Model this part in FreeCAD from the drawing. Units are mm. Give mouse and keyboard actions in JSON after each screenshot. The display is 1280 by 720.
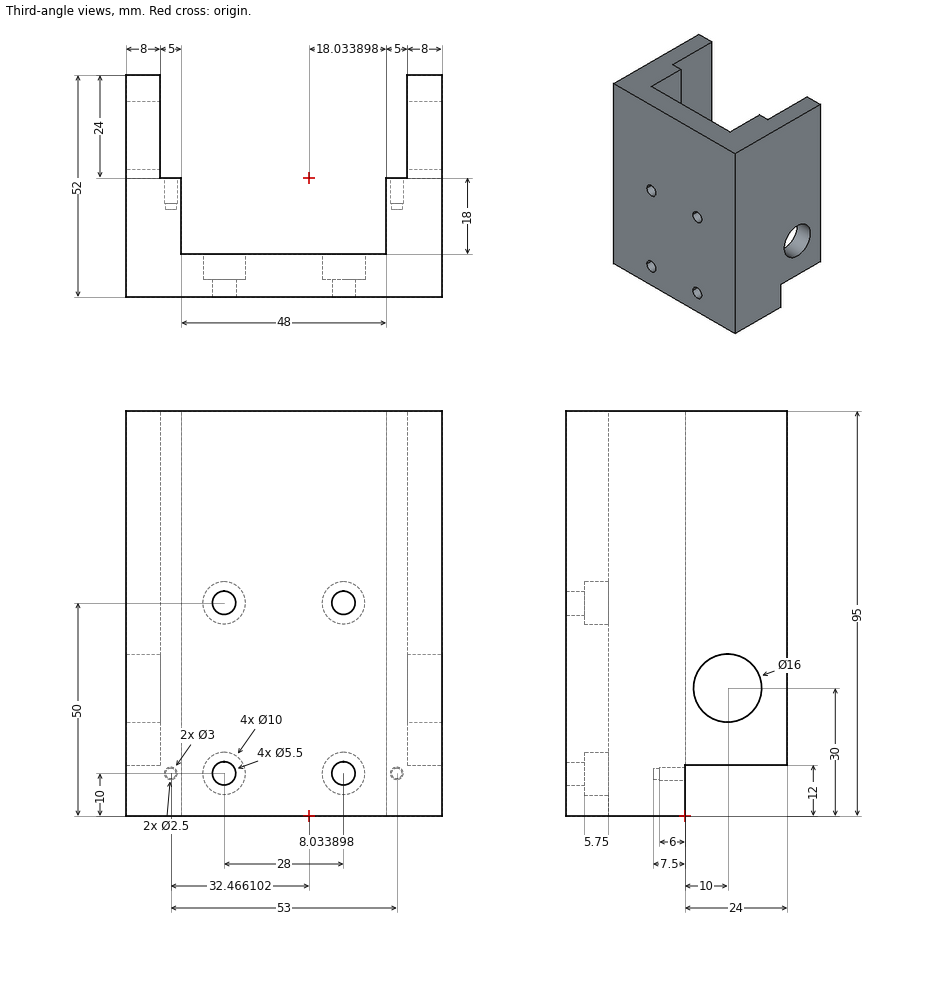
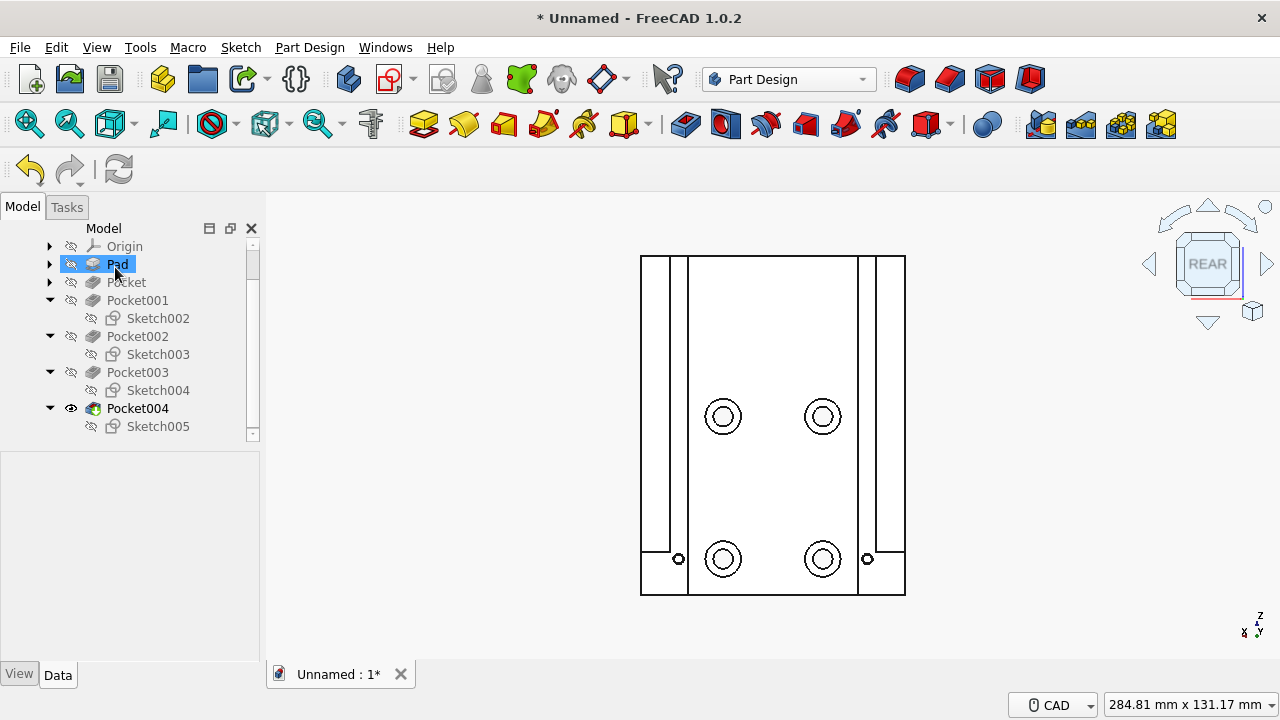
{"action": "key", "text": "6"}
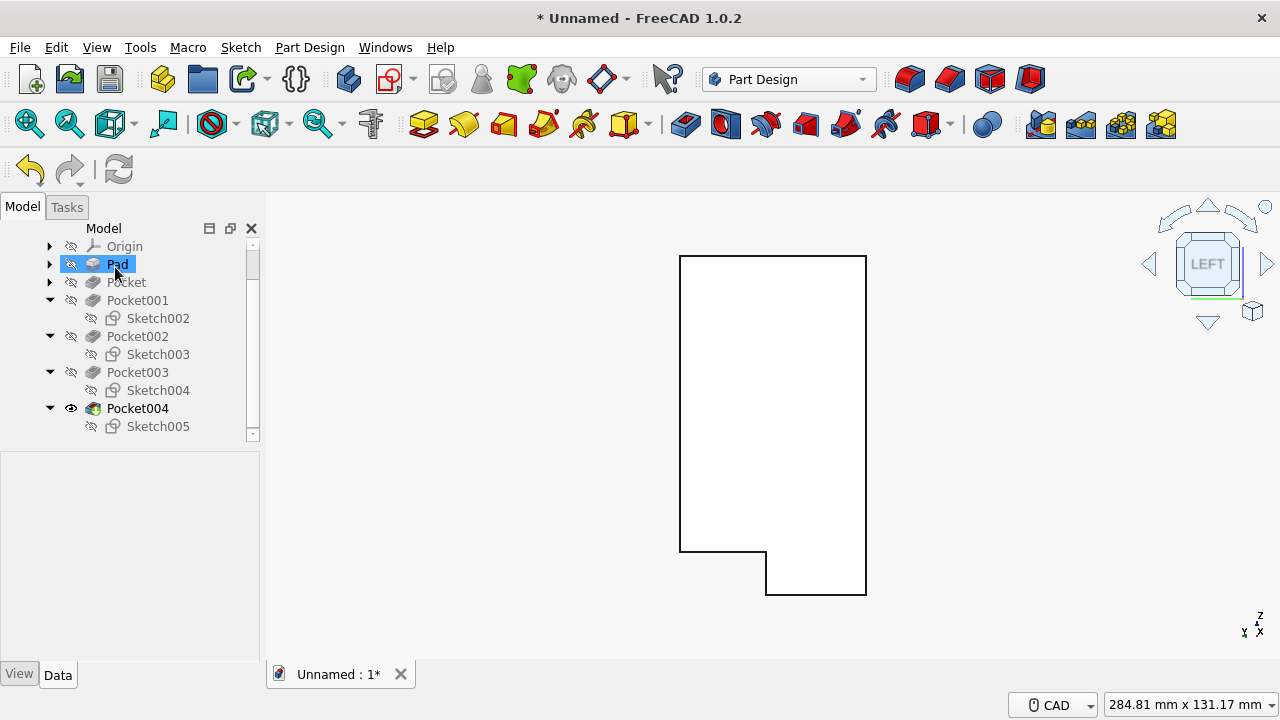
{"action": "left_click", "coordinate": [773, 376]}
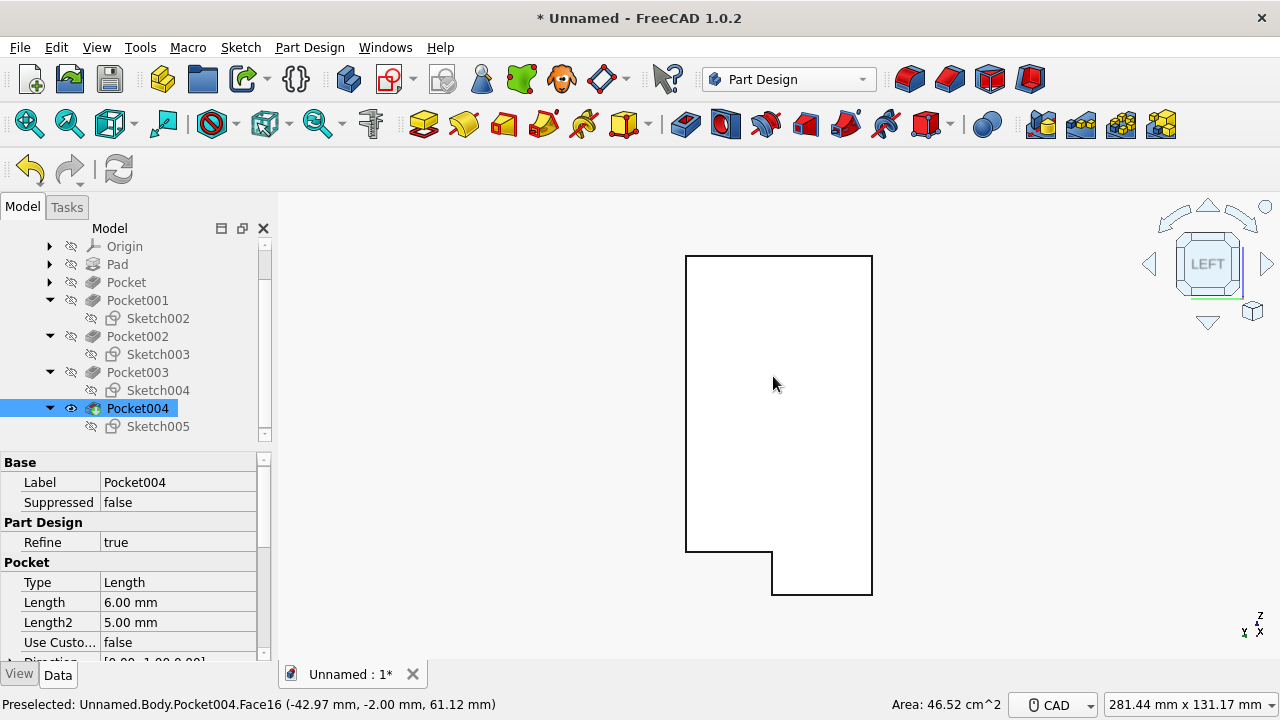
{"action": "left_click", "coordinate": [390, 80]}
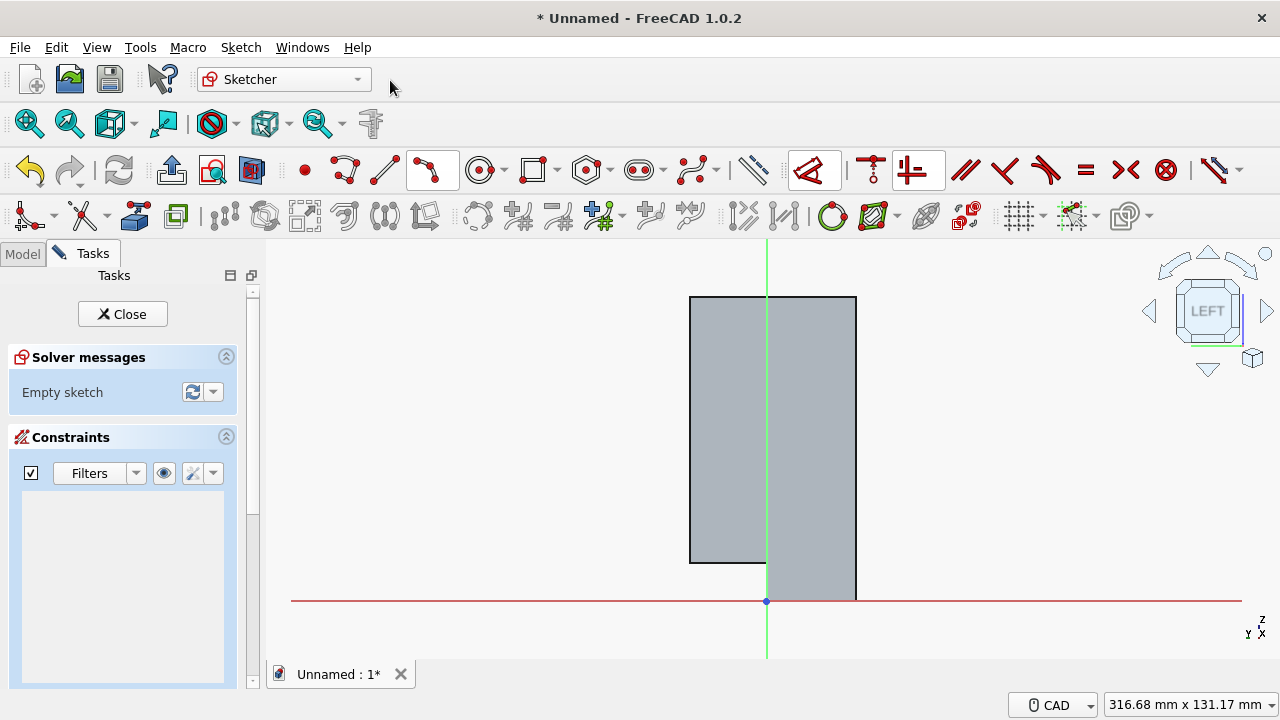
{"action": "scroll", "coordinate": [765, 615], "scroll_direction": "up", "scroll_amount": 4}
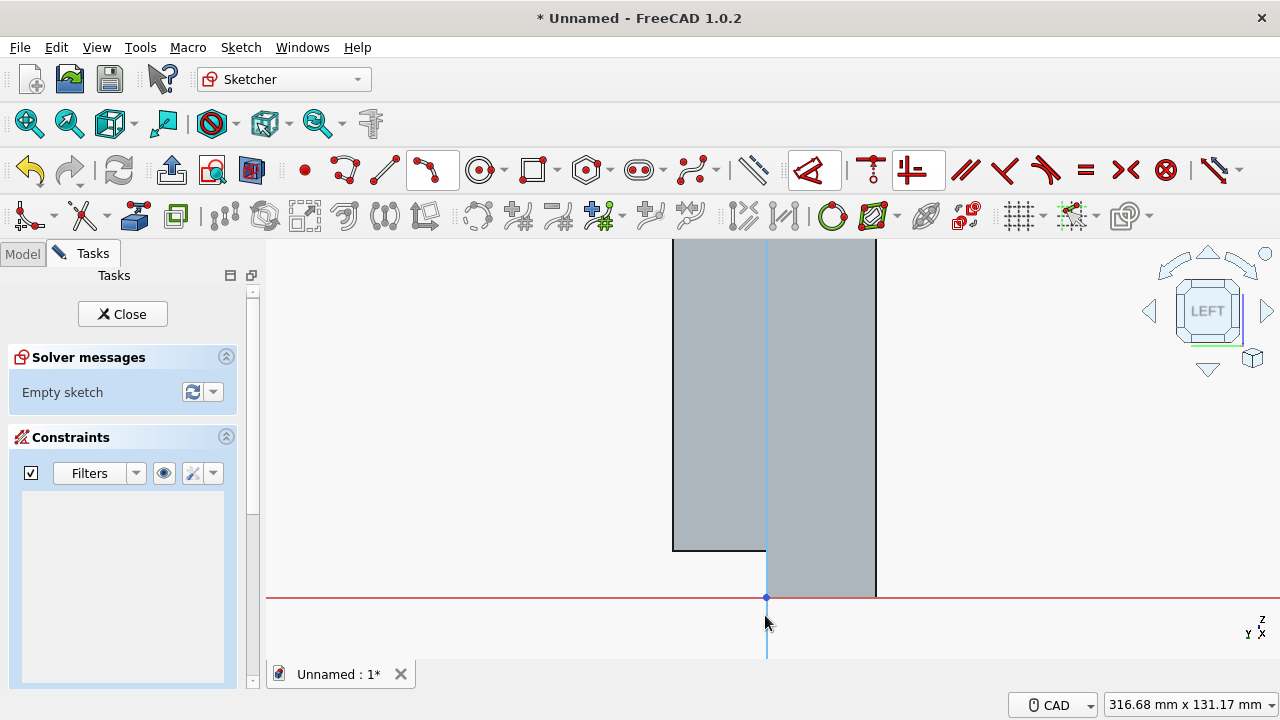
{"action": "left_click", "coordinate": [480, 170]}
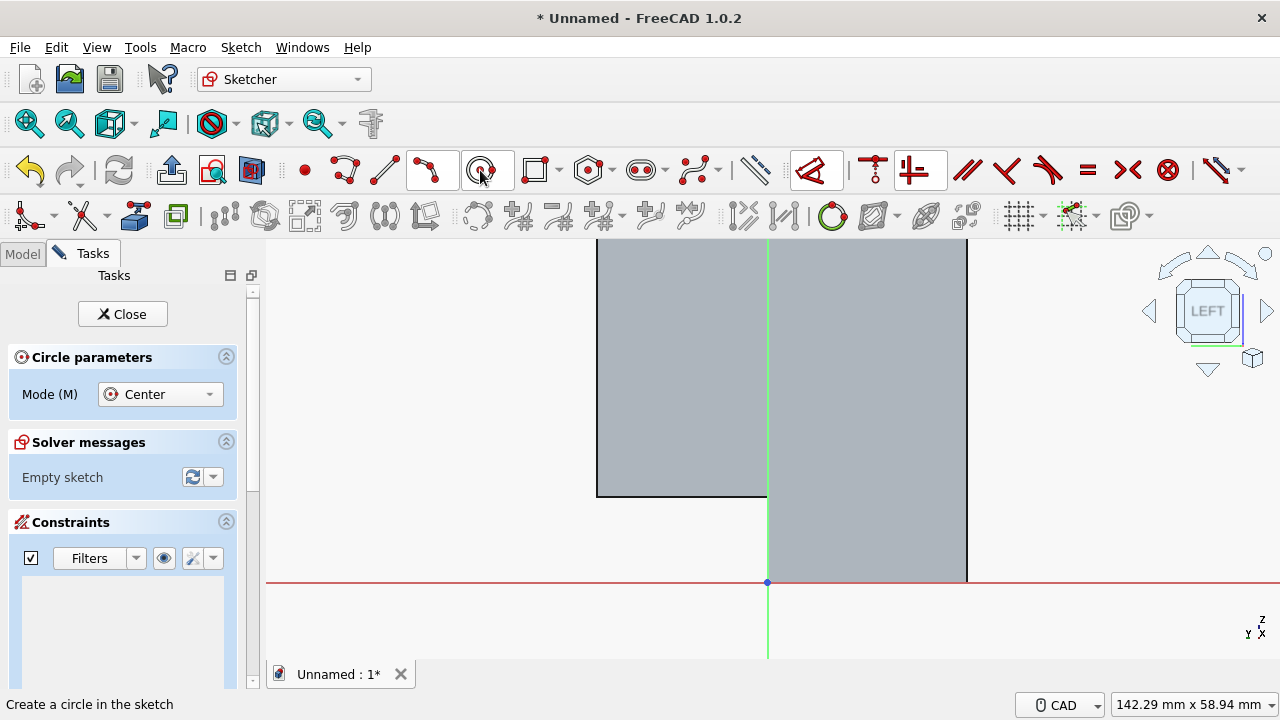
{"action": "left_click", "coordinate": [697, 369]}
{"action": "left_click", "coordinate": [737, 329]}
{"action": "key", "text": "Escape"}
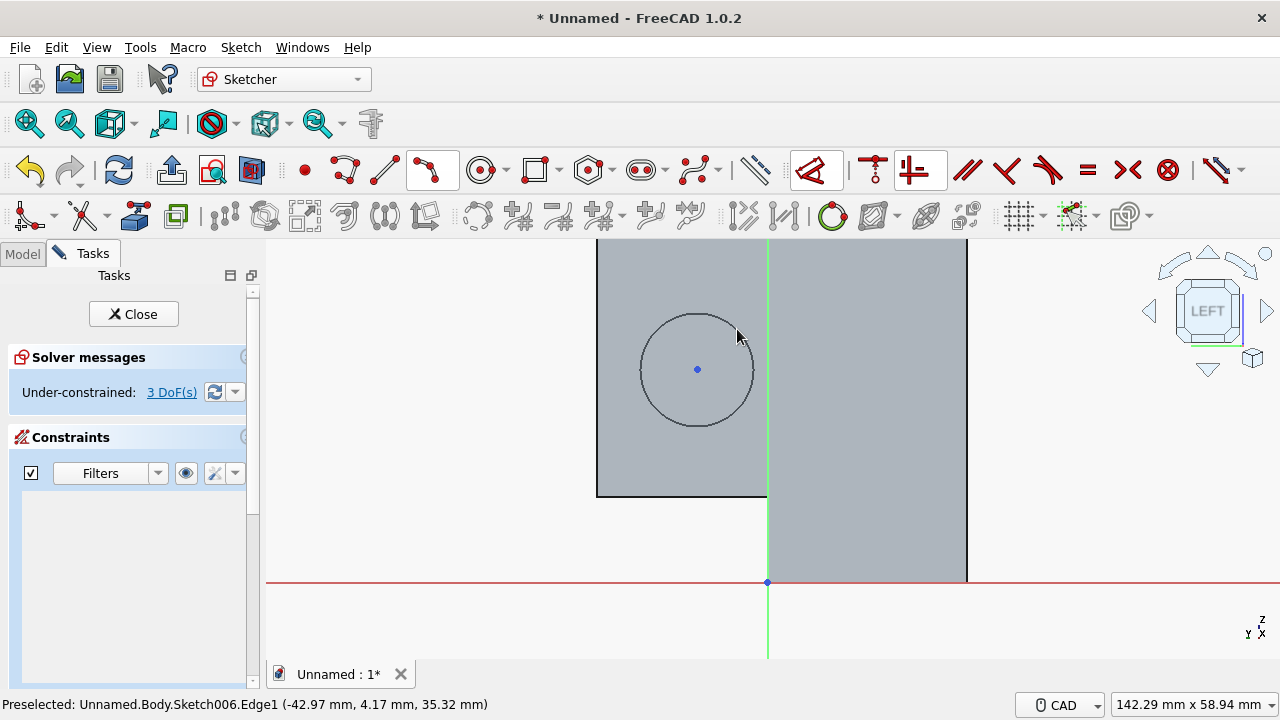
{"action": "left_click", "coordinate": [737, 330]}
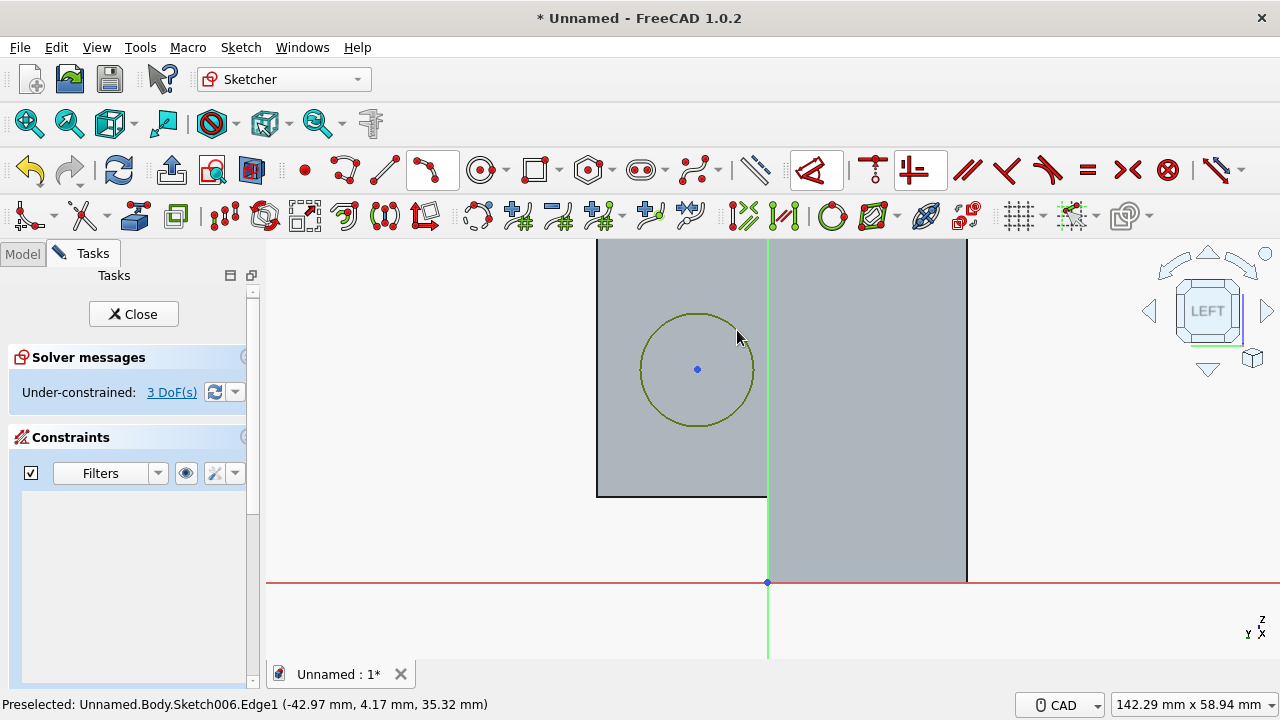
{"action": "key", "text": "k o"}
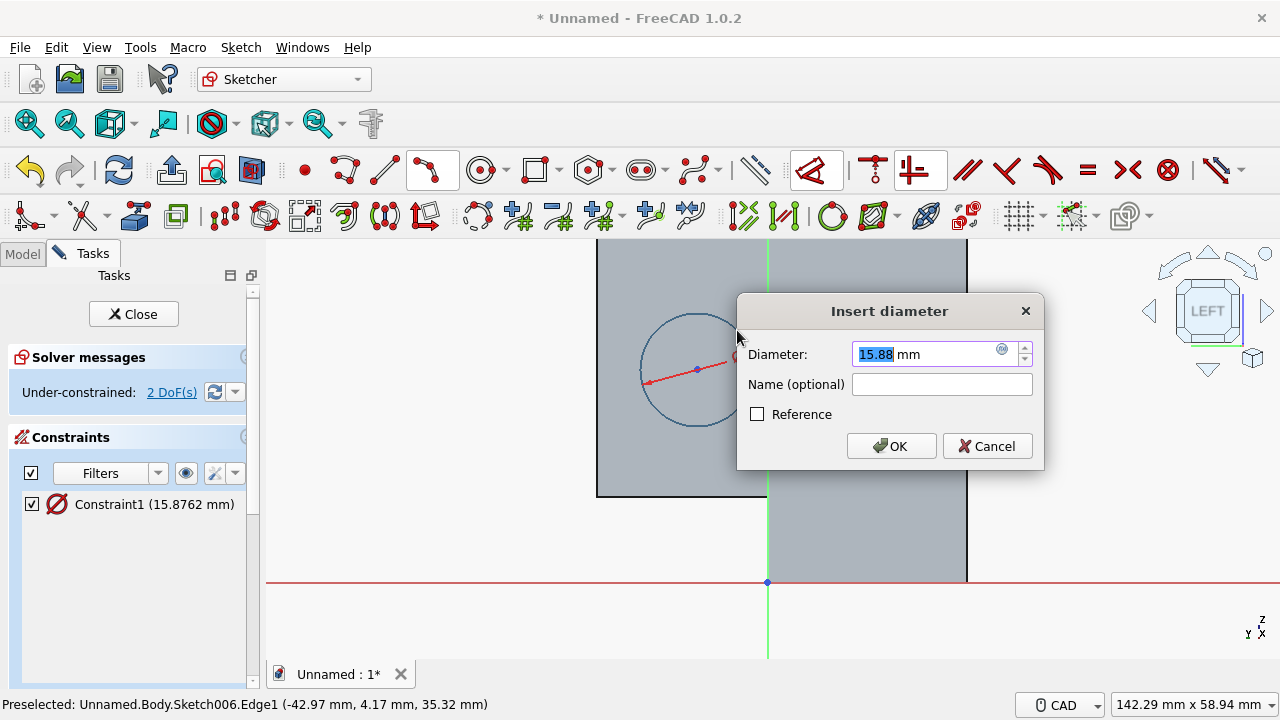
{"action": "type", "text": "16"}
{"action": "key", "text": "Return"}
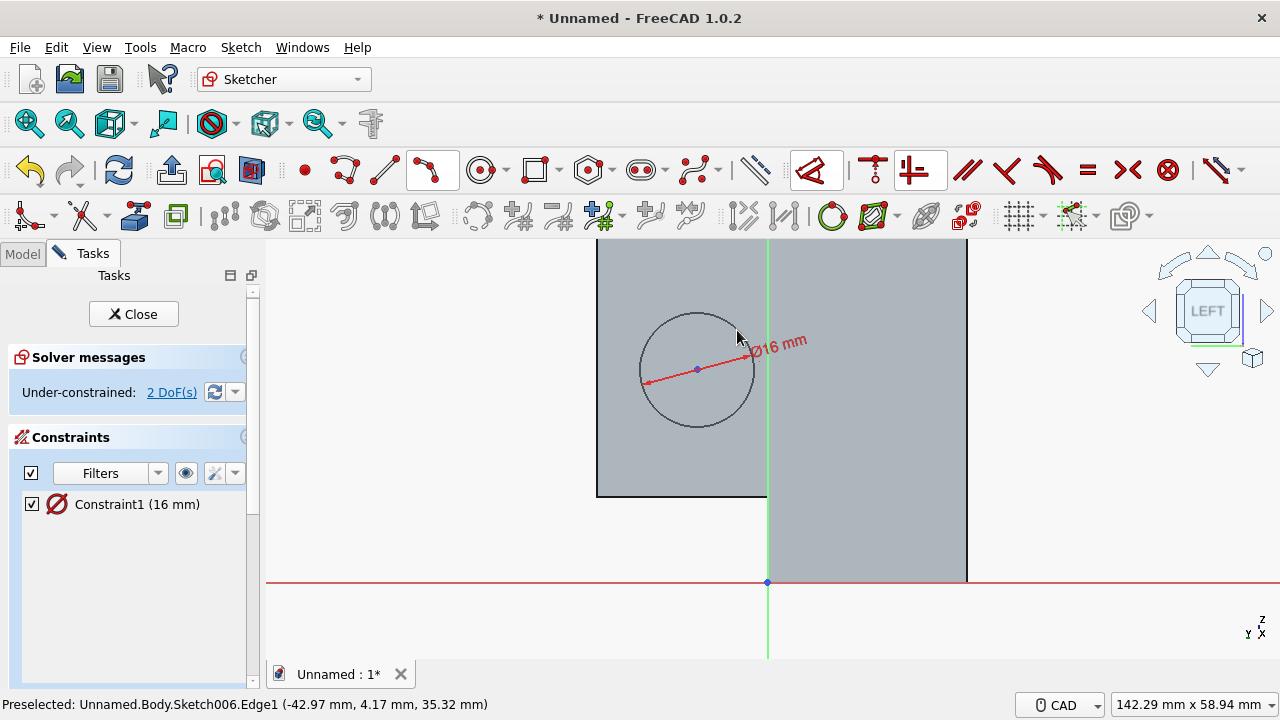
{"action": "left_click", "coordinate": [697, 370]}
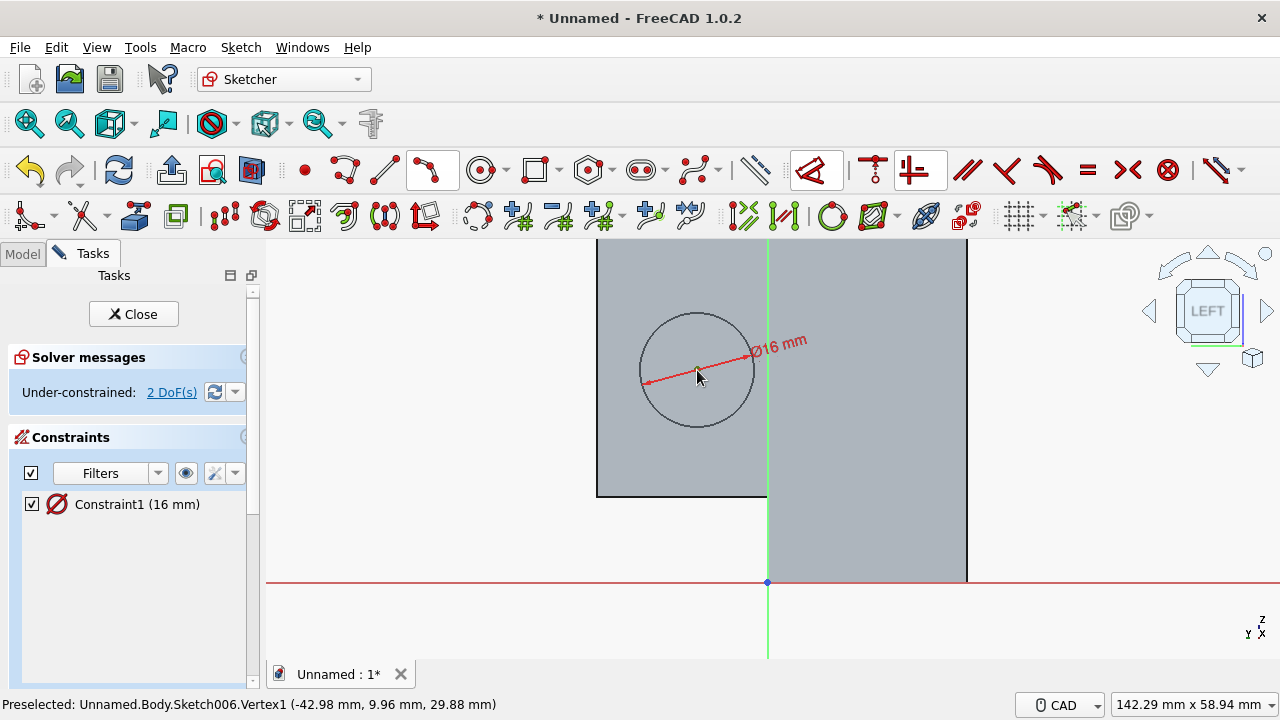
{"action": "key", "text": "l"}